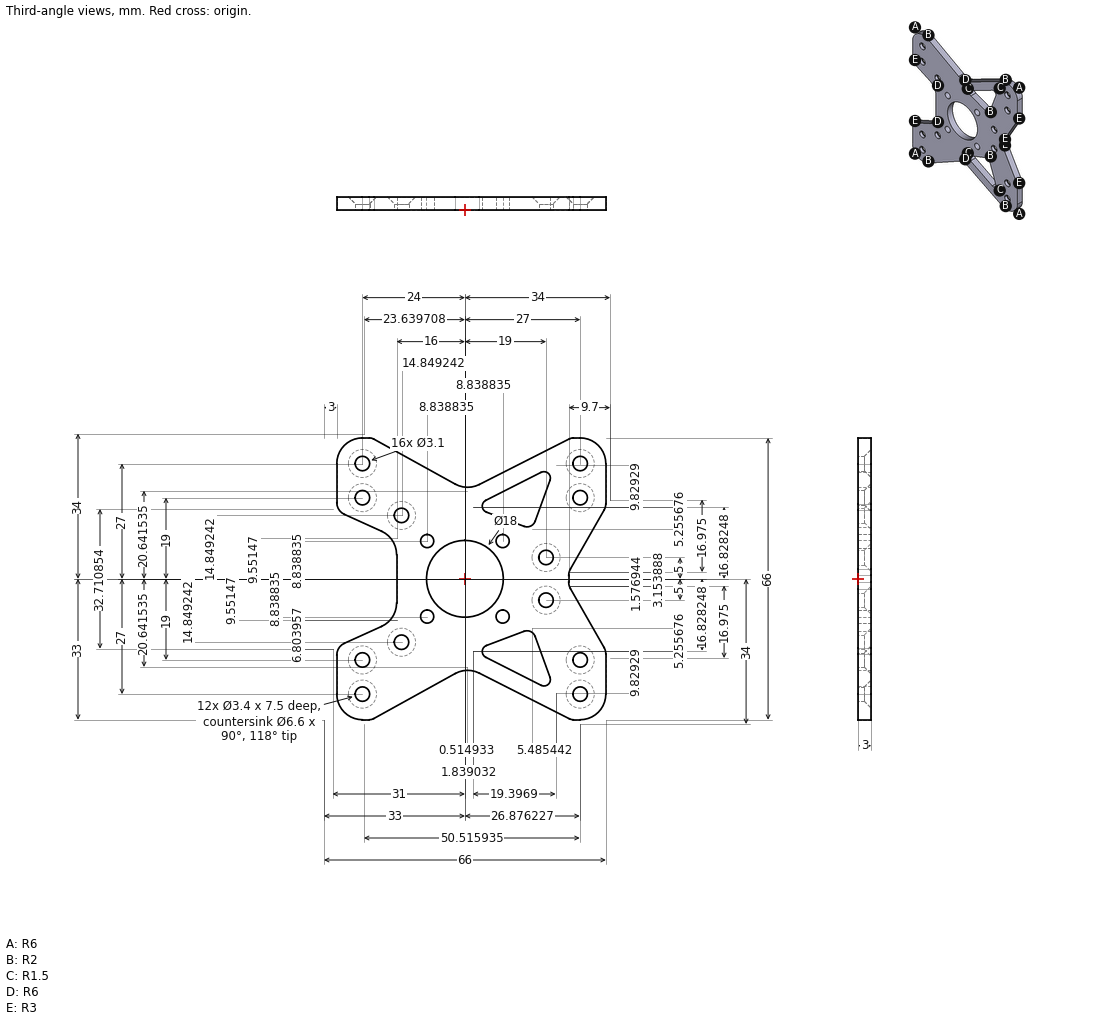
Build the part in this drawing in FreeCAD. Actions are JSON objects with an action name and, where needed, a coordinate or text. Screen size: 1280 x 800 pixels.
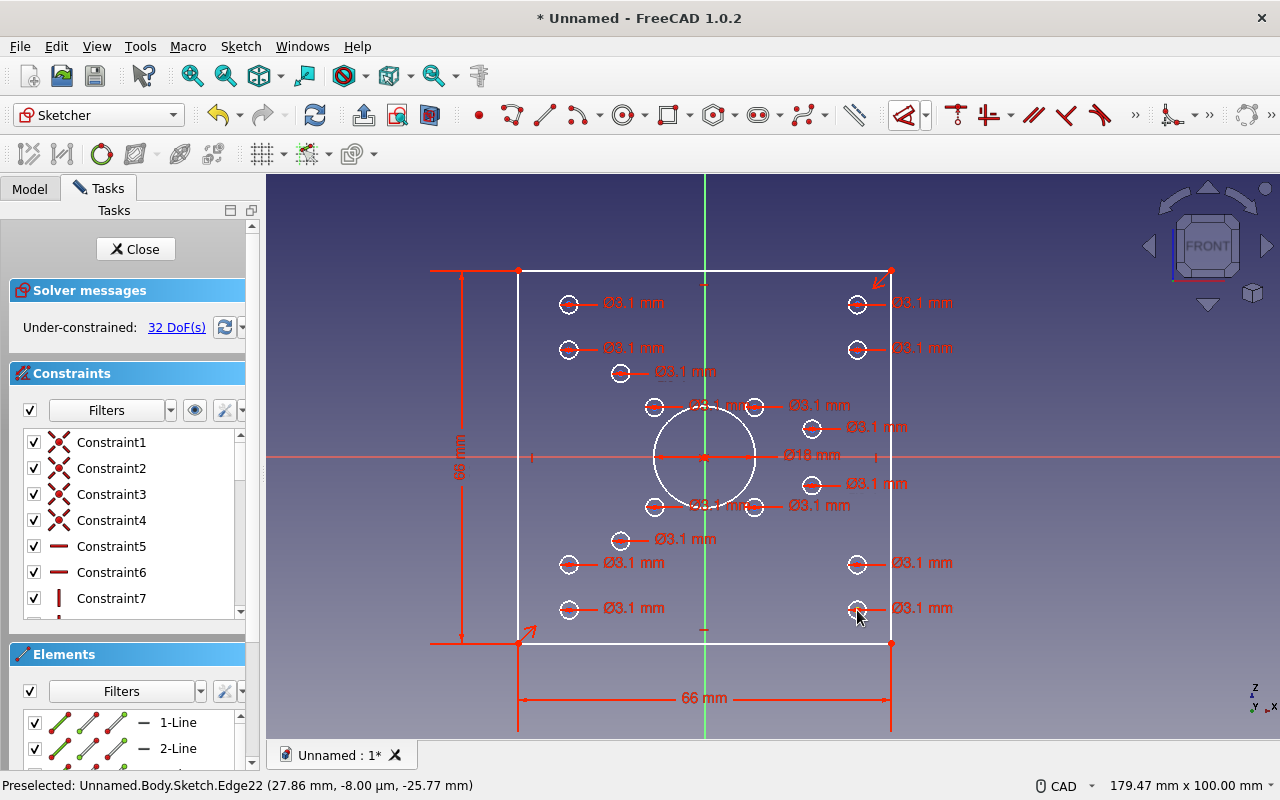
{"action": "left_click", "coordinate": [569, 305]}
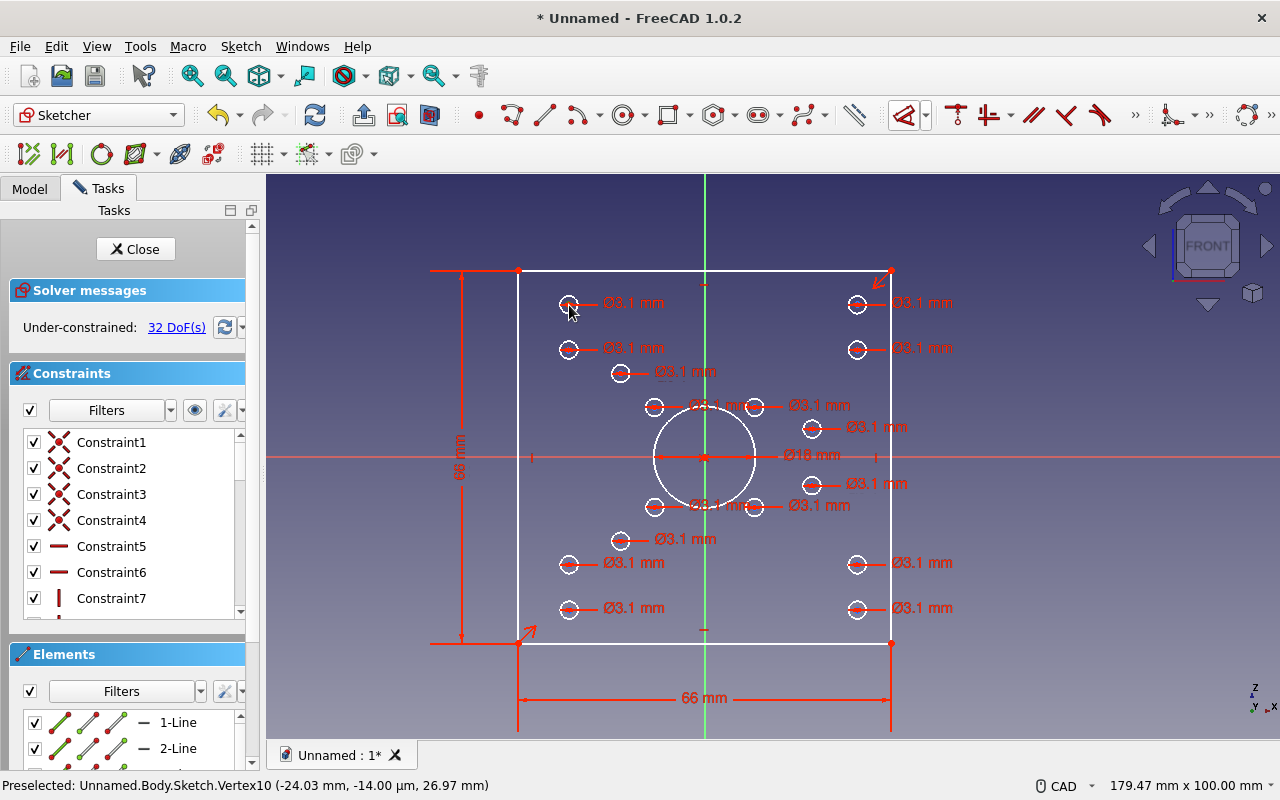
{"action": "left_click", "coordinate": [569, 350]}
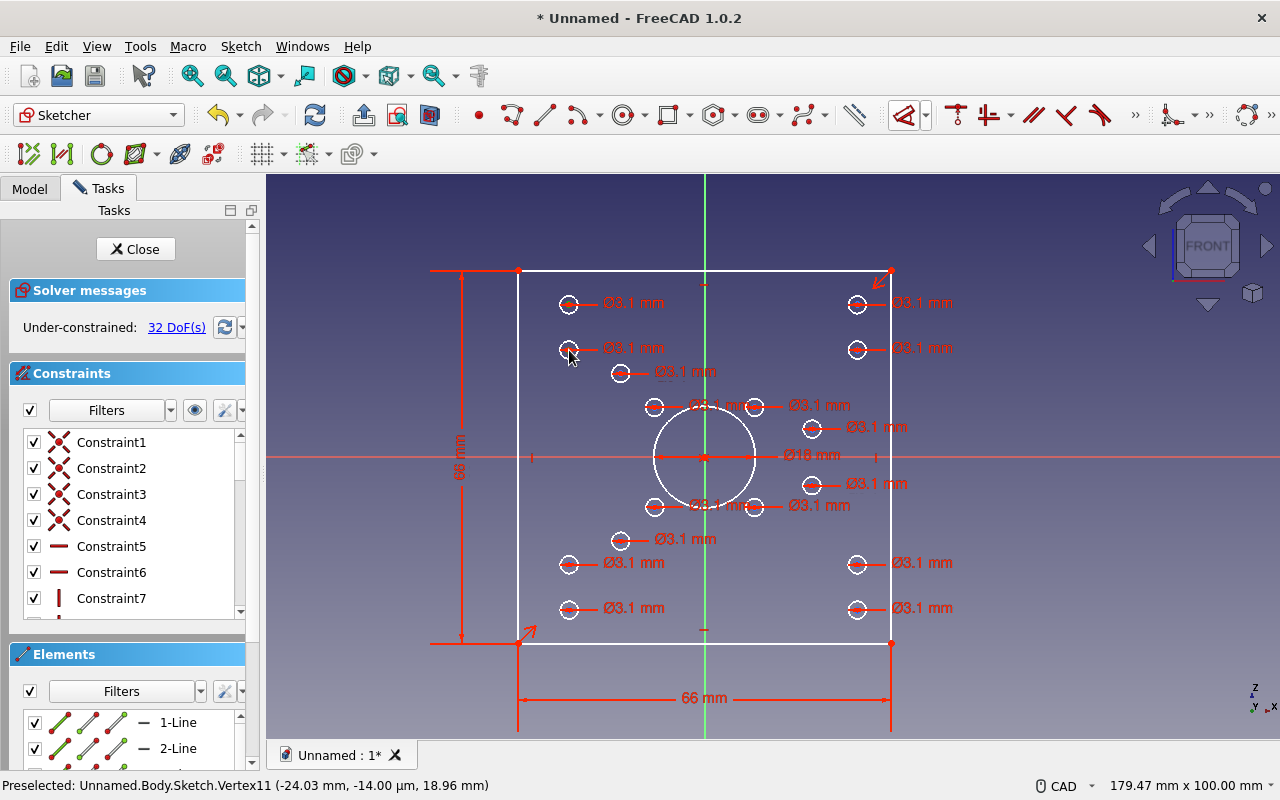
{"action": "left_click", "coordinate": [1010, 116]}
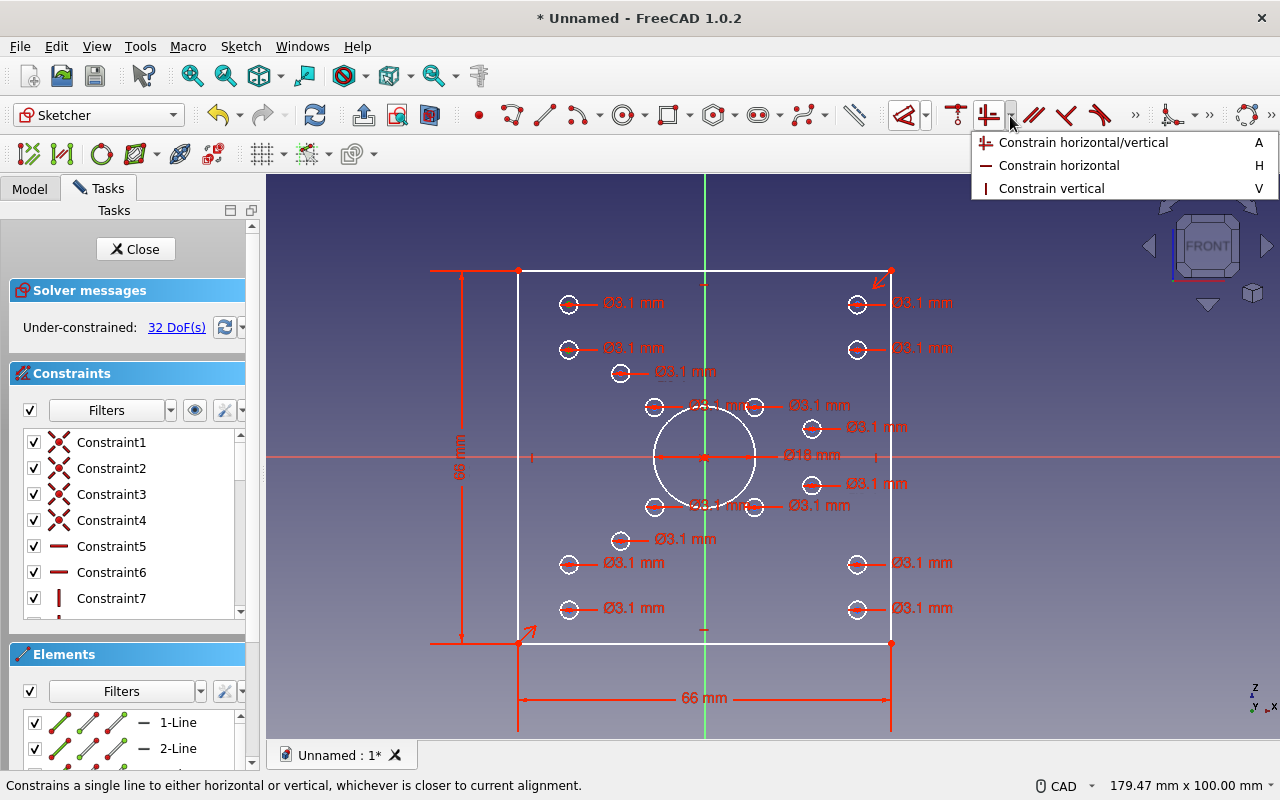
{"action": "left_click", "coordinate": [1125, 188]}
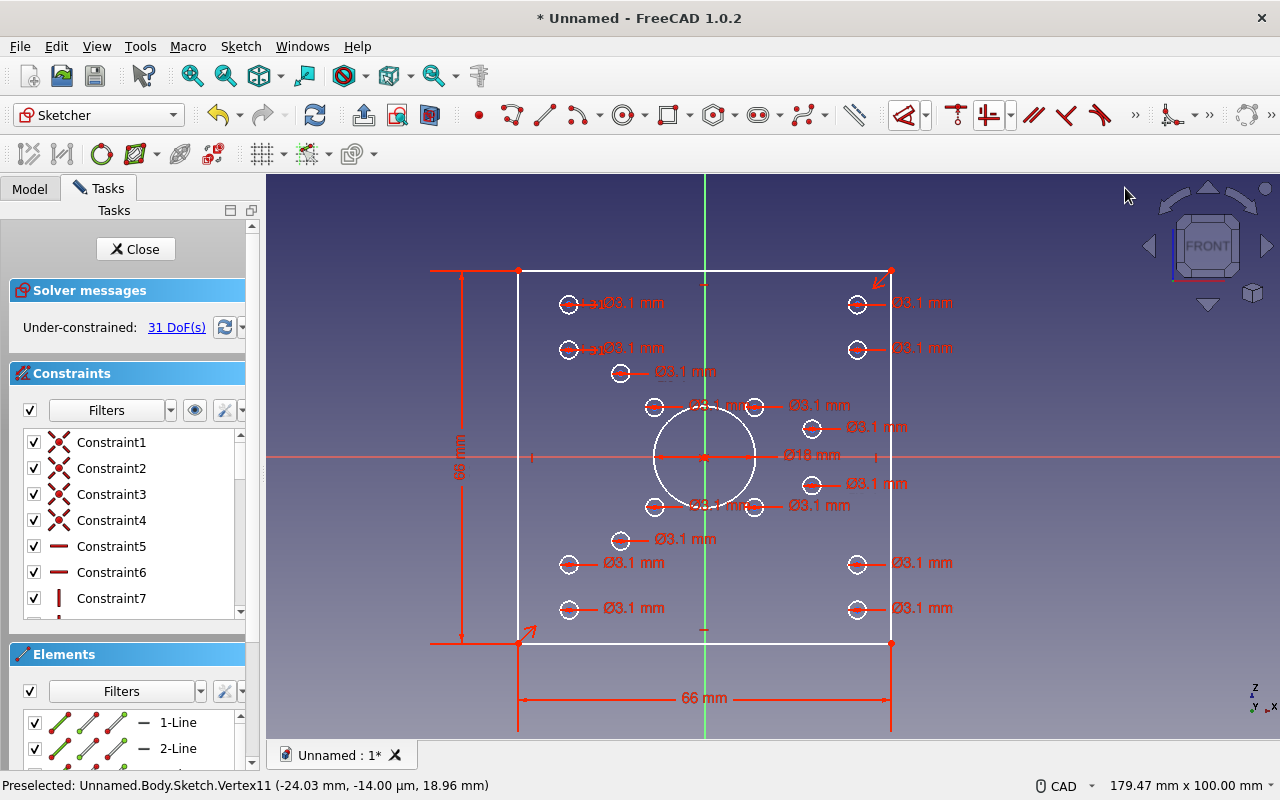
{"action": "left_click", "coordinate": [569, 305]}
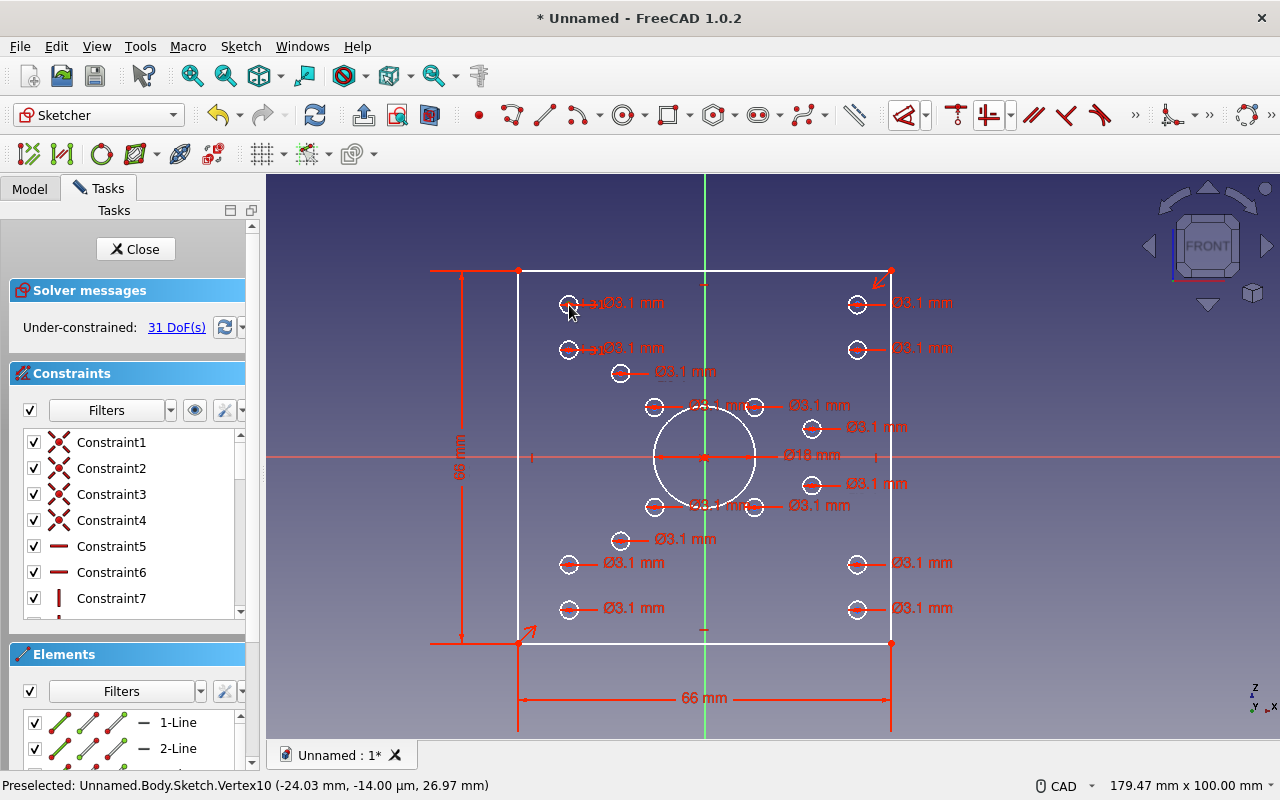
{"action": "left_click", "coordinate": [857, 305]}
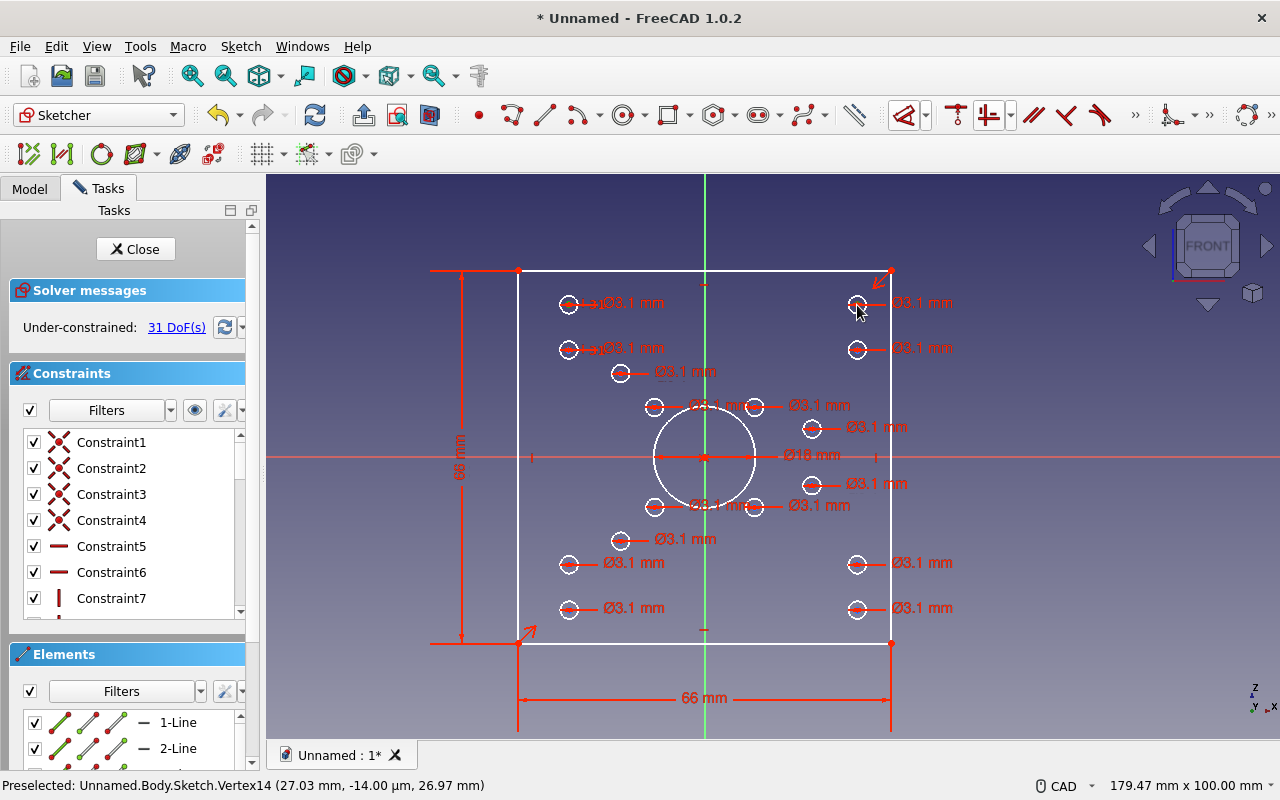
{"action": "left_click", "coordinate": [1010, 116]}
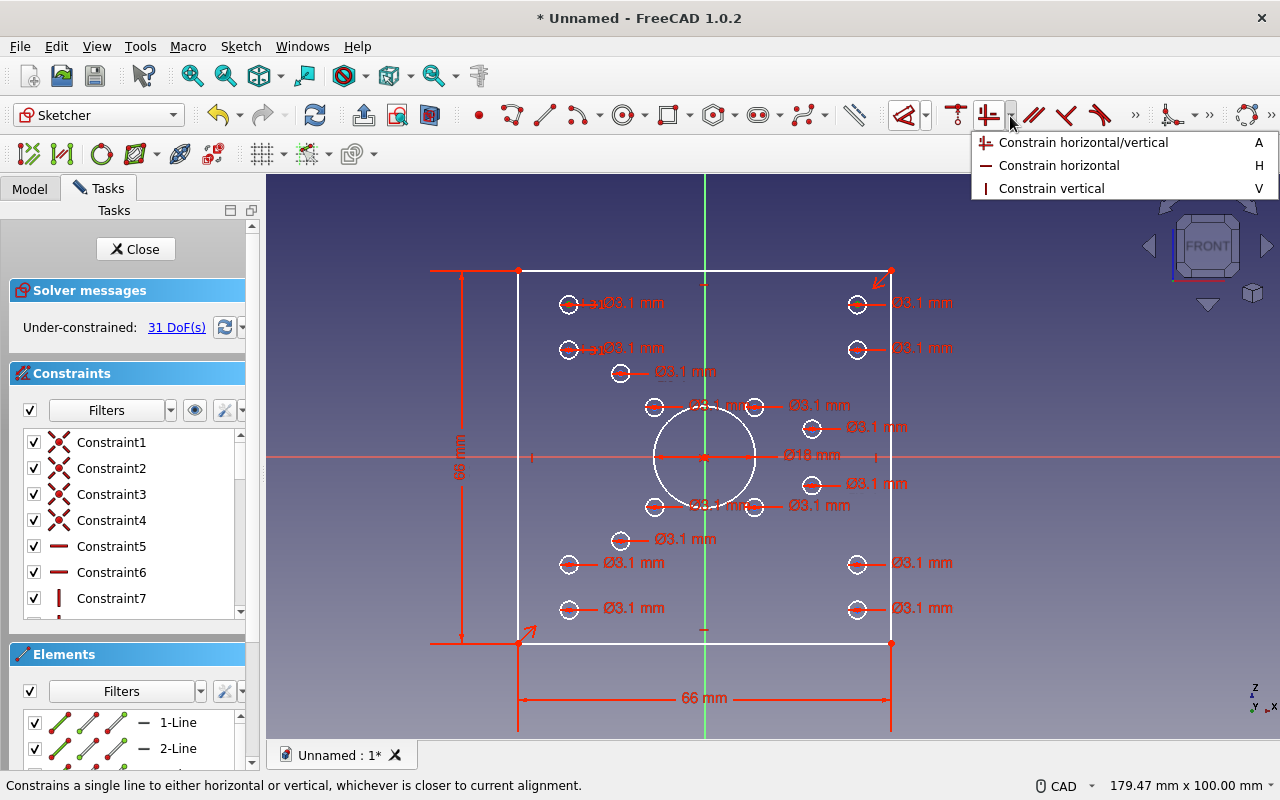
{"action": "left_click", "coordinate": [1125, 166]}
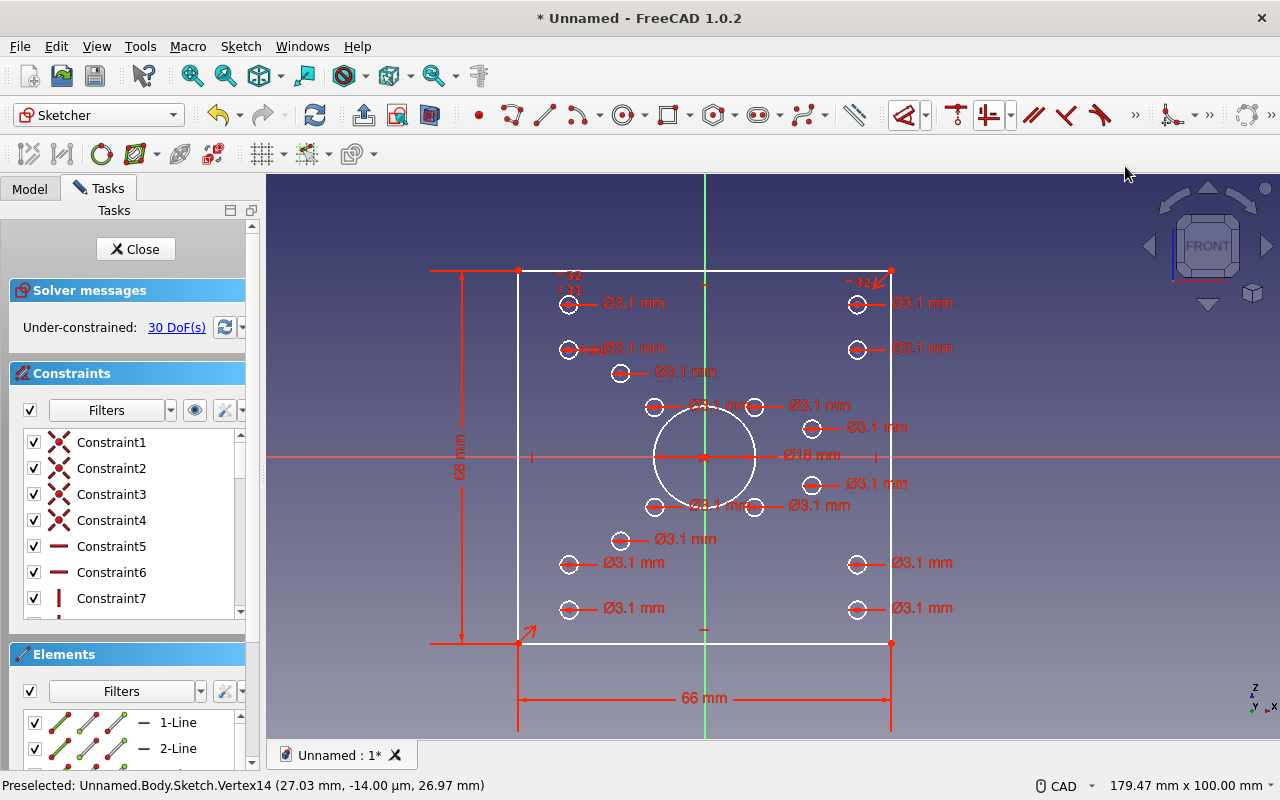
{"action": "left_click", "coordinate": [857, 305]}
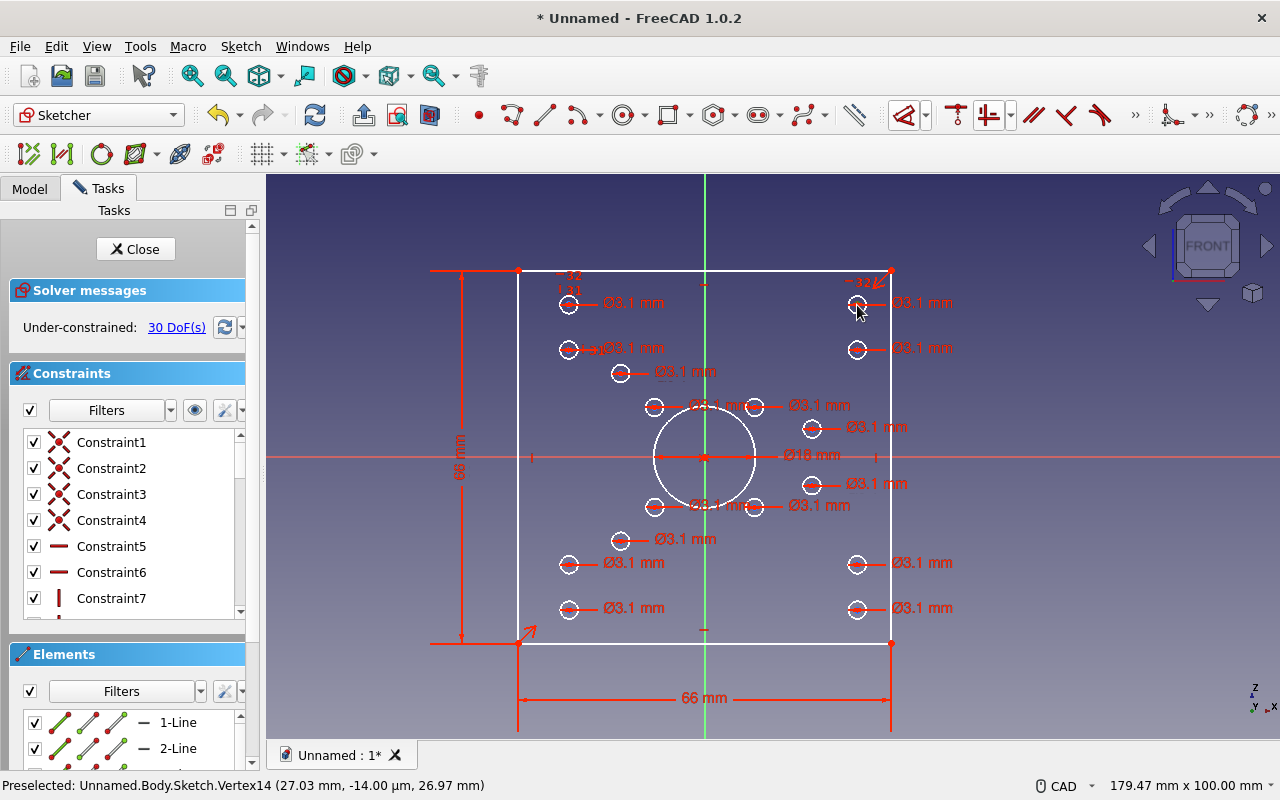
{"action": "left_click", "coordinate": [857, 350]}